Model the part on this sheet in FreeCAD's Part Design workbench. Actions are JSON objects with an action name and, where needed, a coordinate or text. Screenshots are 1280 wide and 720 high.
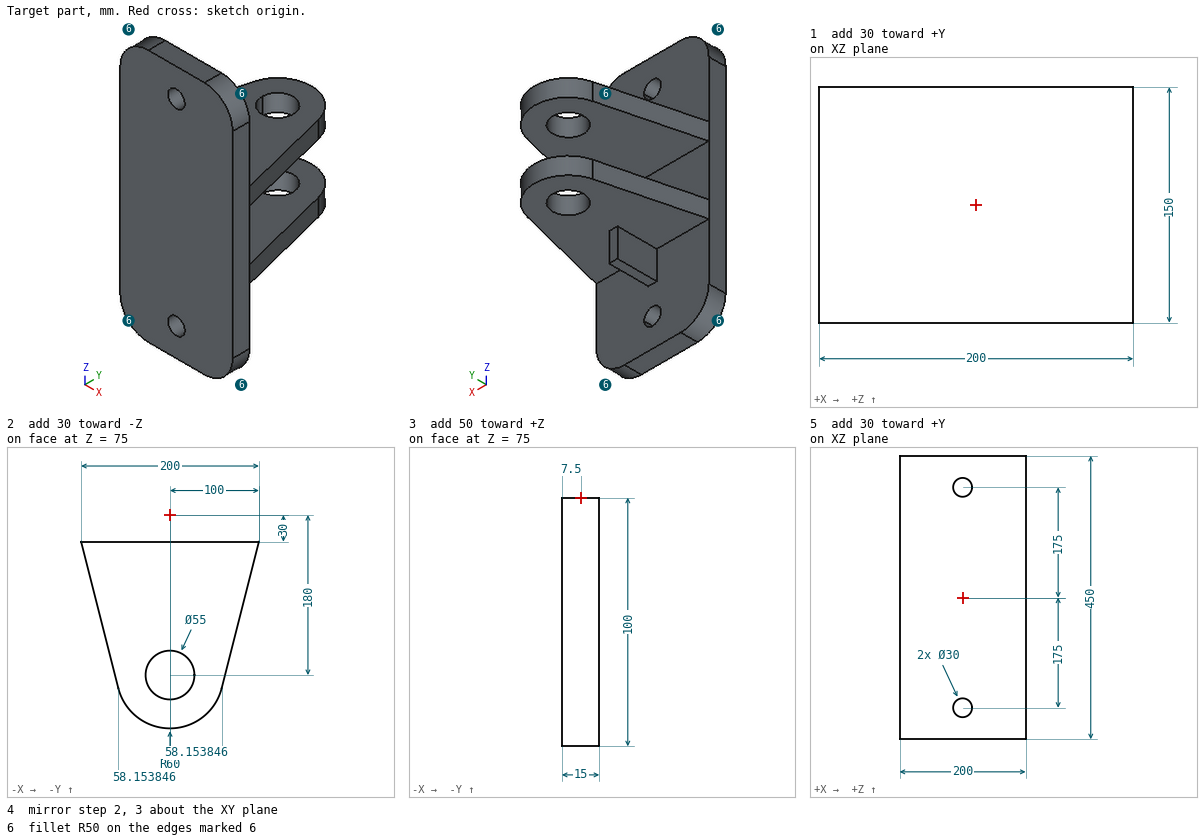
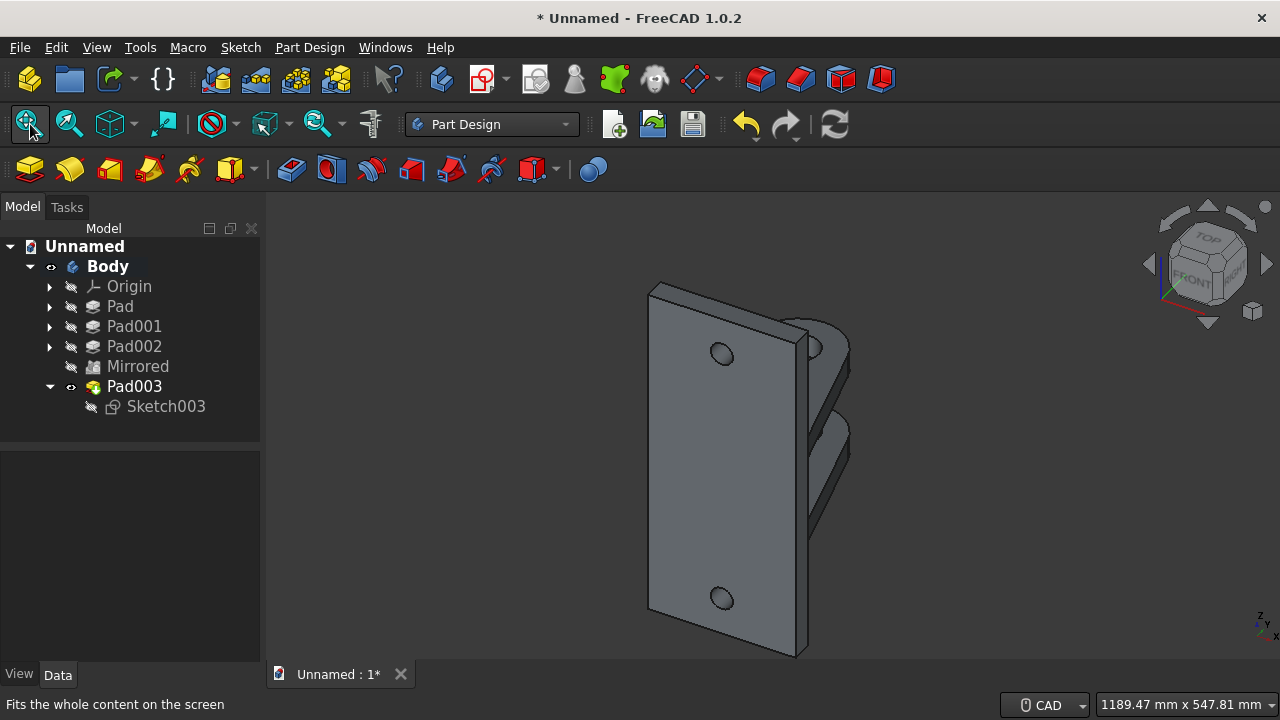
{"action": "left_click", "coordinate": [802, 336]}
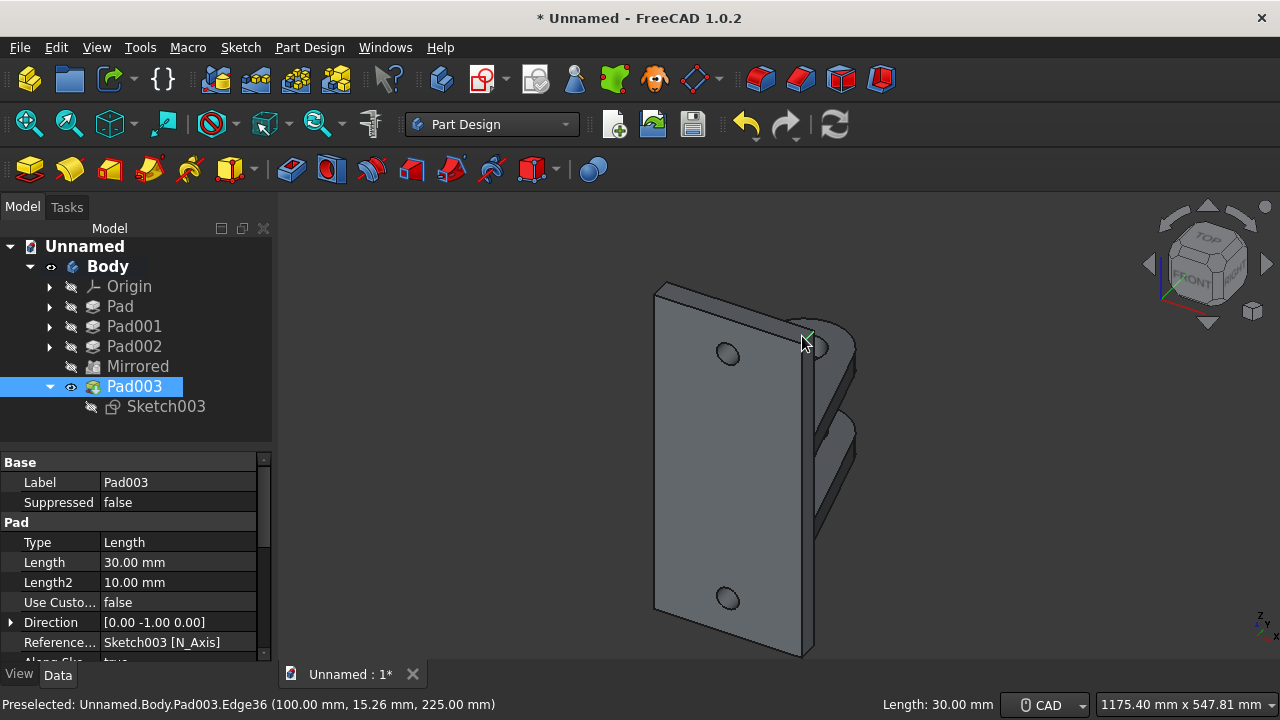
{"action": "key", "text": "0"}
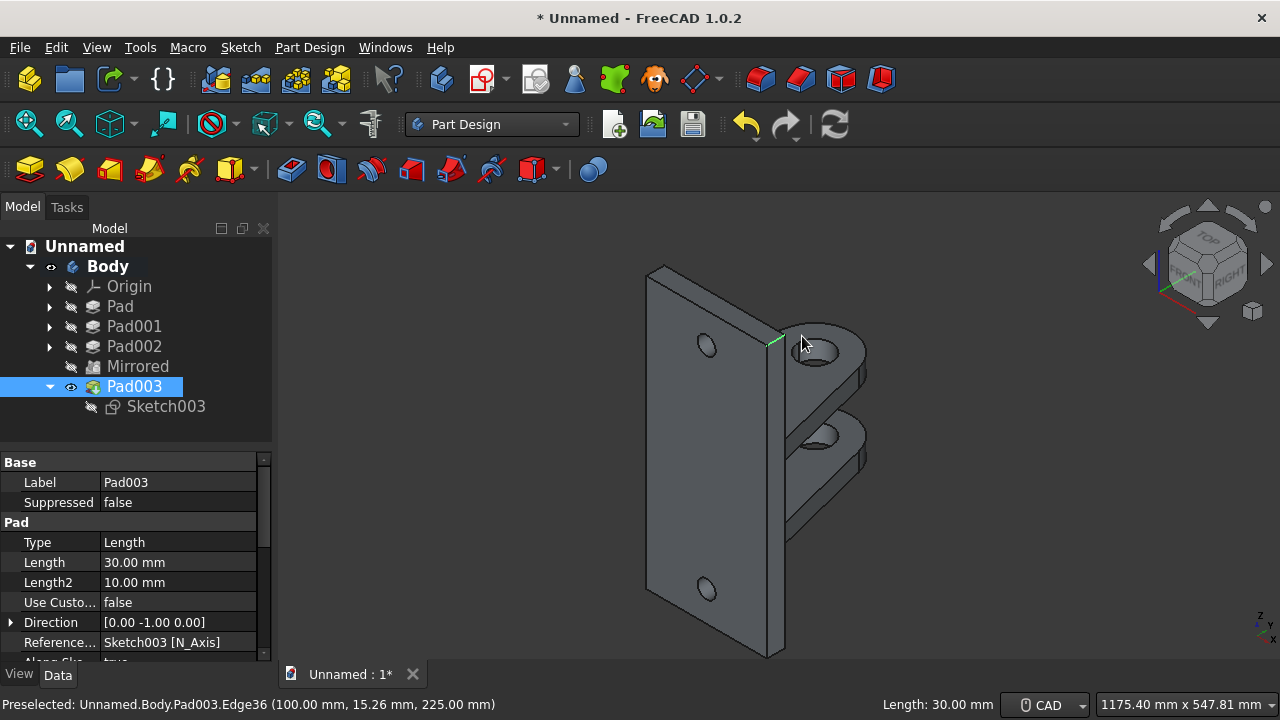
{"action": "key", "text": "v f"}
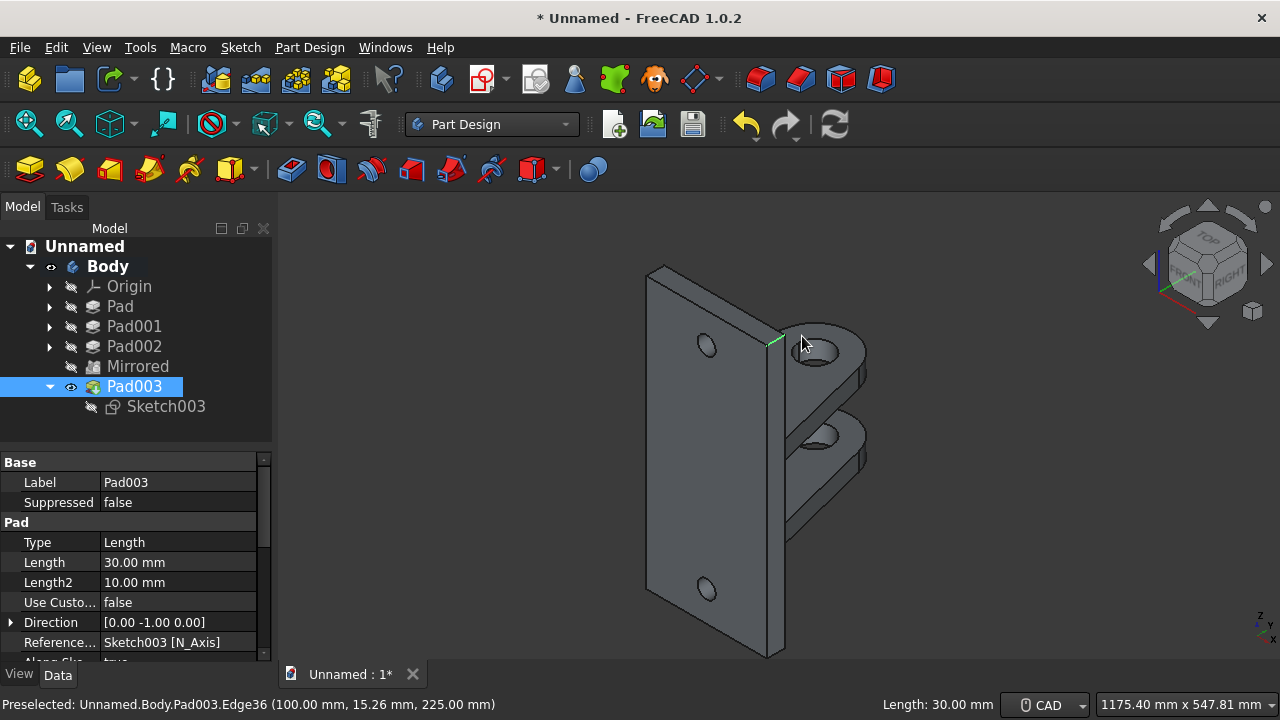
{"action": "key", "text": "2"}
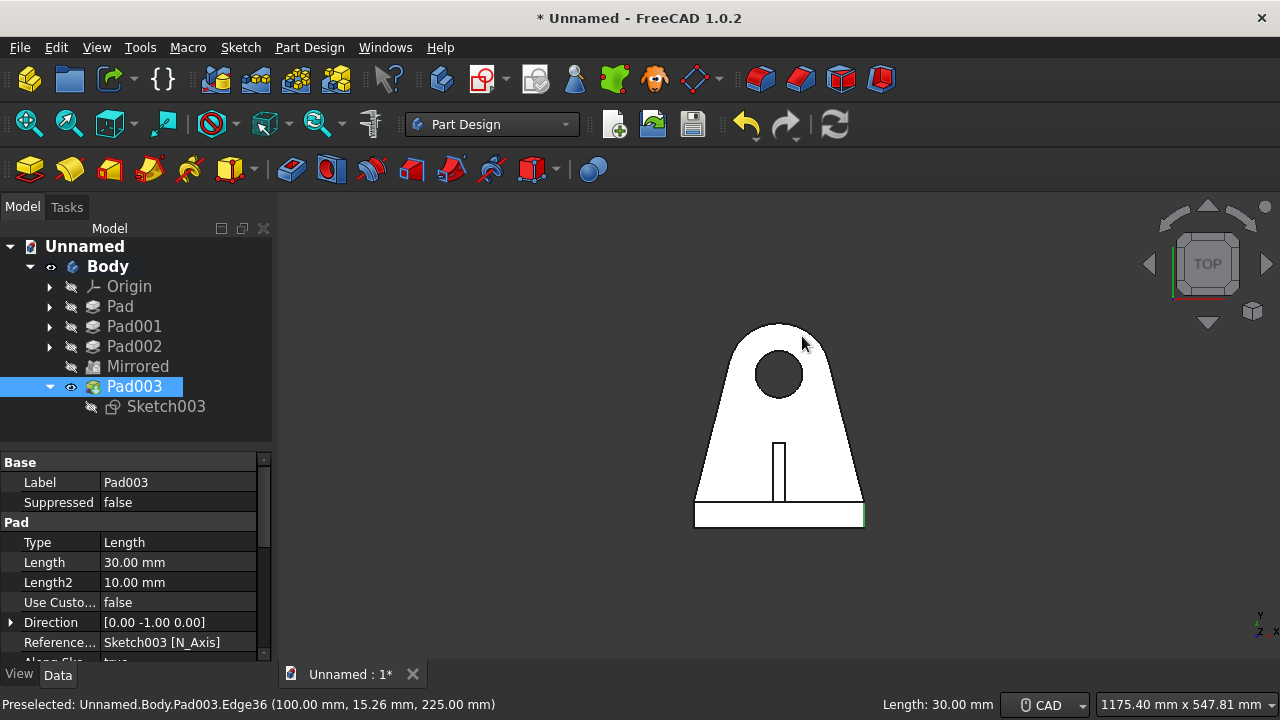
{"action": "key", "text": "v f"}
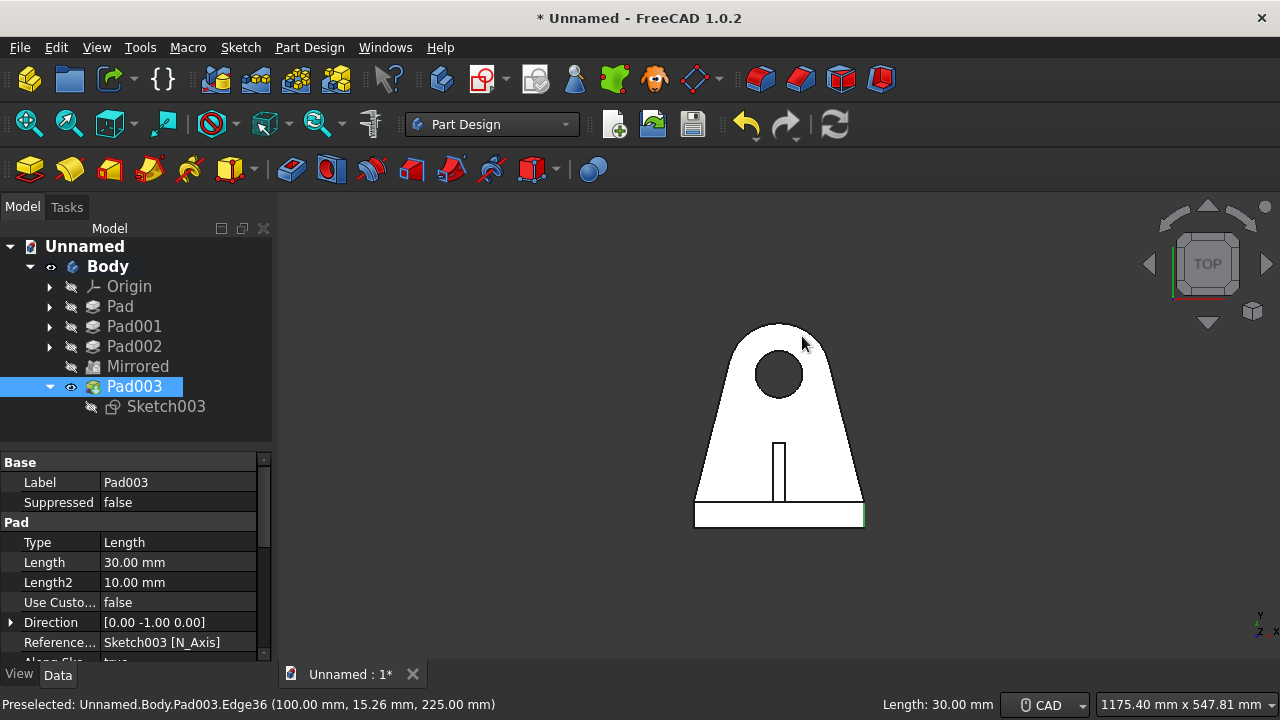
{"action": "left_click", "coordinate": [694, 514], "text": "ctrl"}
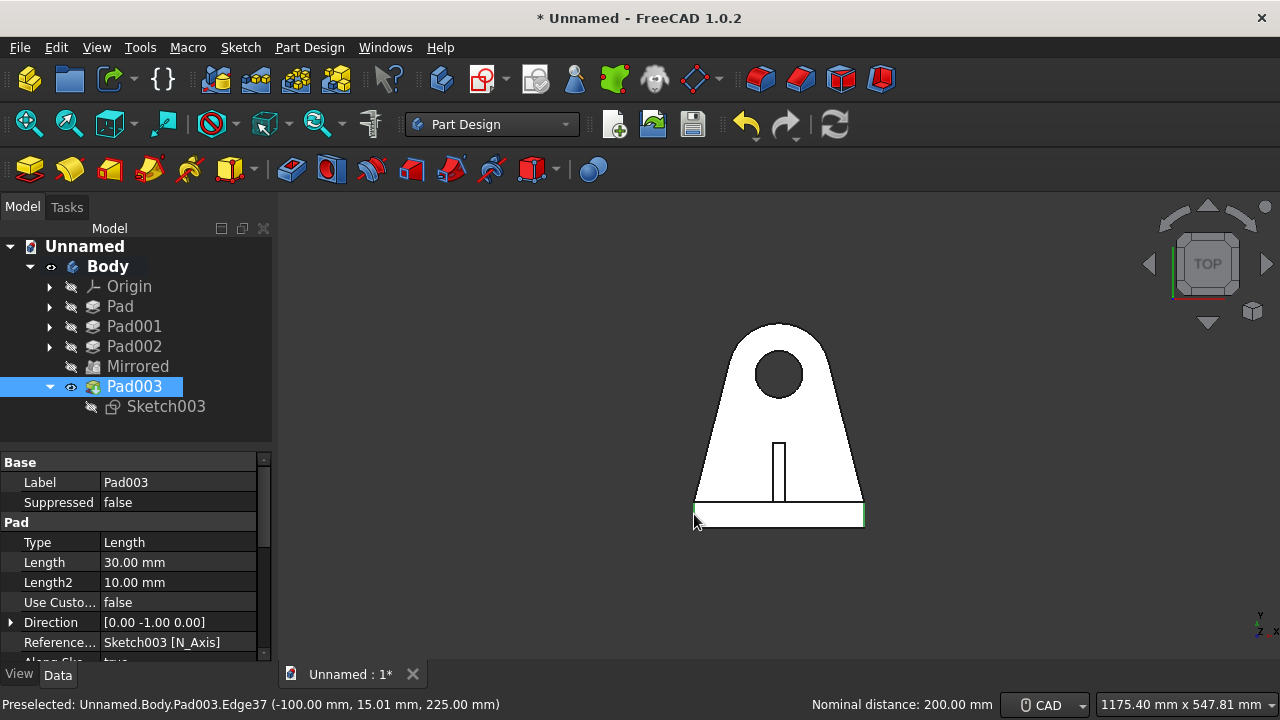
{"action": "key", "text": "1"}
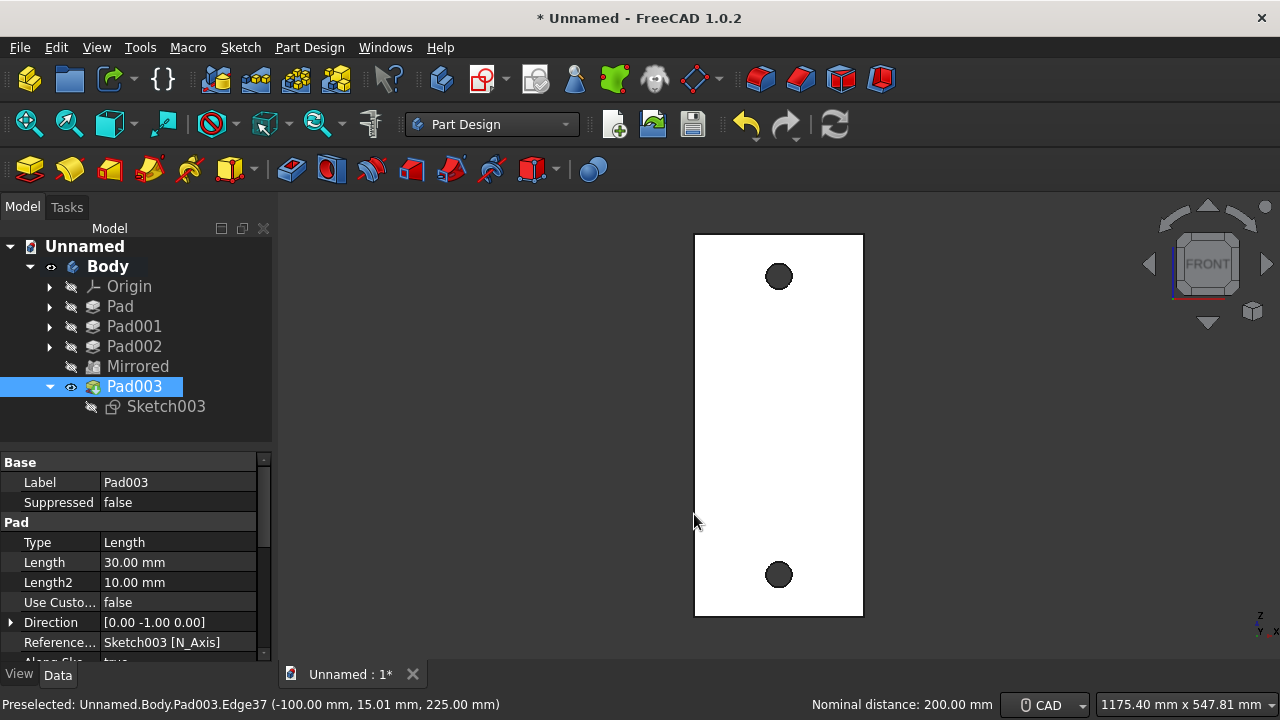
{"action": "key", "text": "3"}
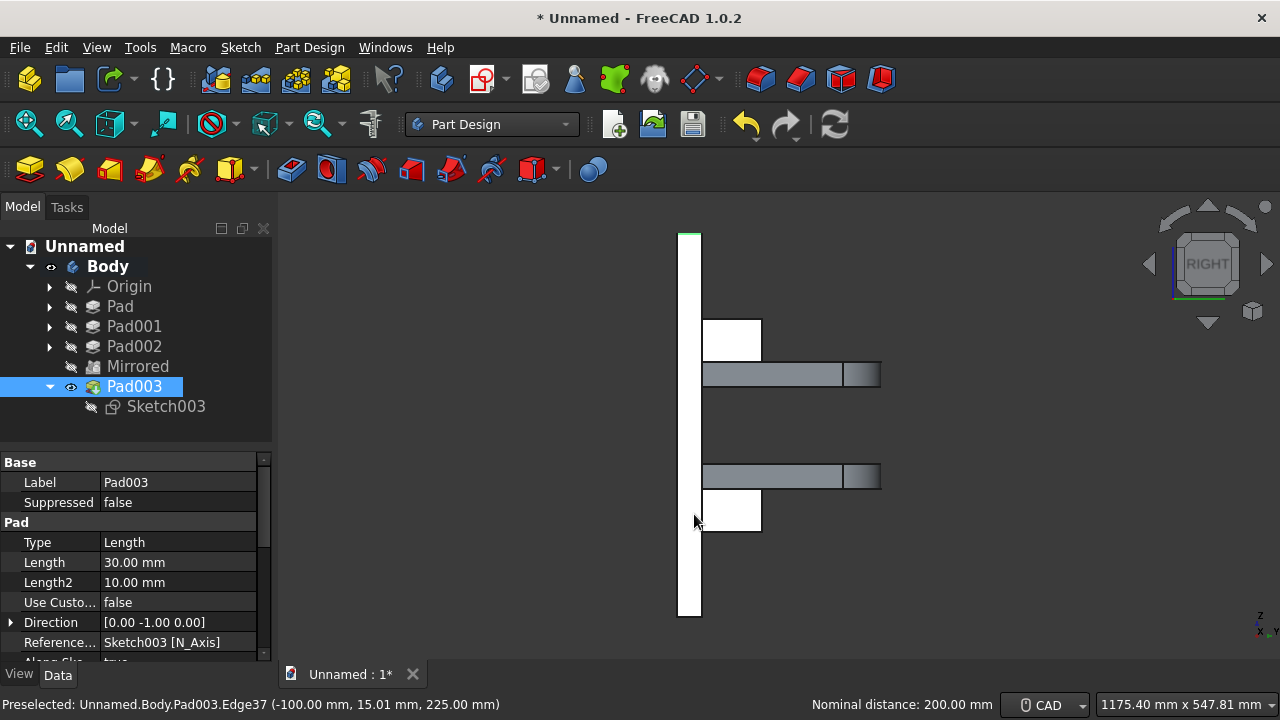
{"action": "left_click", "coordinate": [689, 616], "text": "ctrl"}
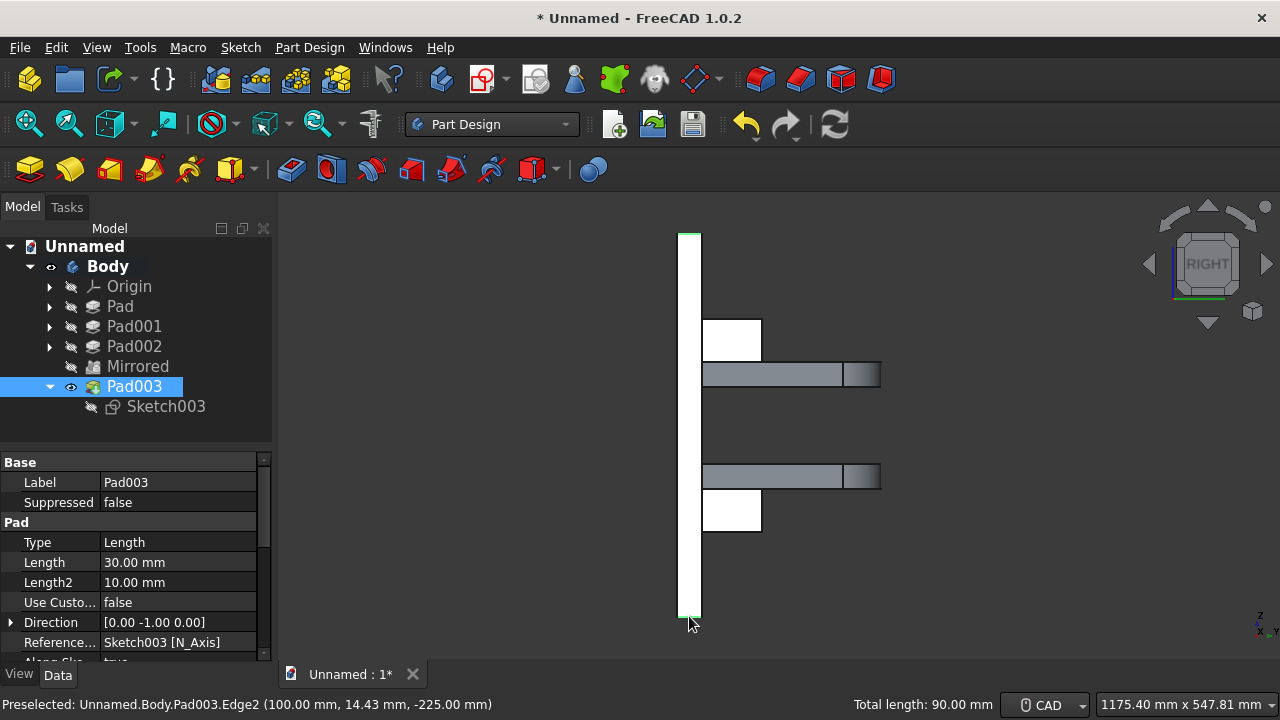
{"action": "key", "text": "5"}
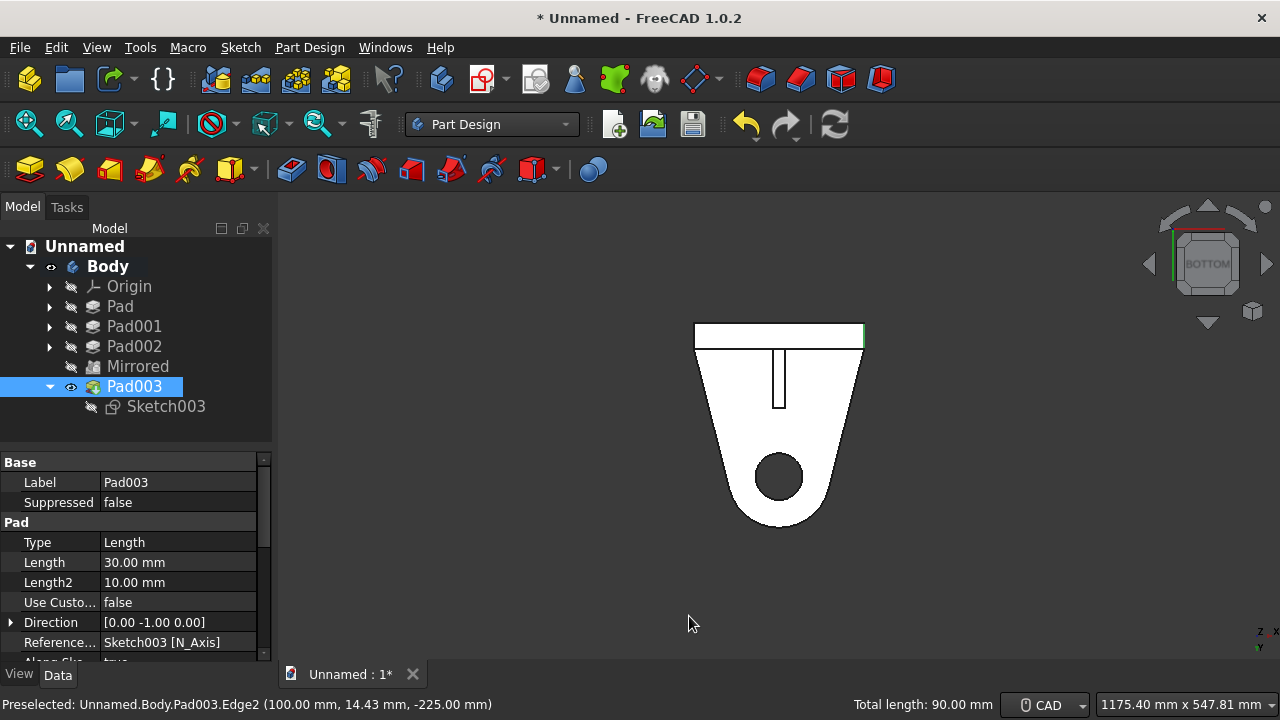
{"action": "key", "text": "v f"}